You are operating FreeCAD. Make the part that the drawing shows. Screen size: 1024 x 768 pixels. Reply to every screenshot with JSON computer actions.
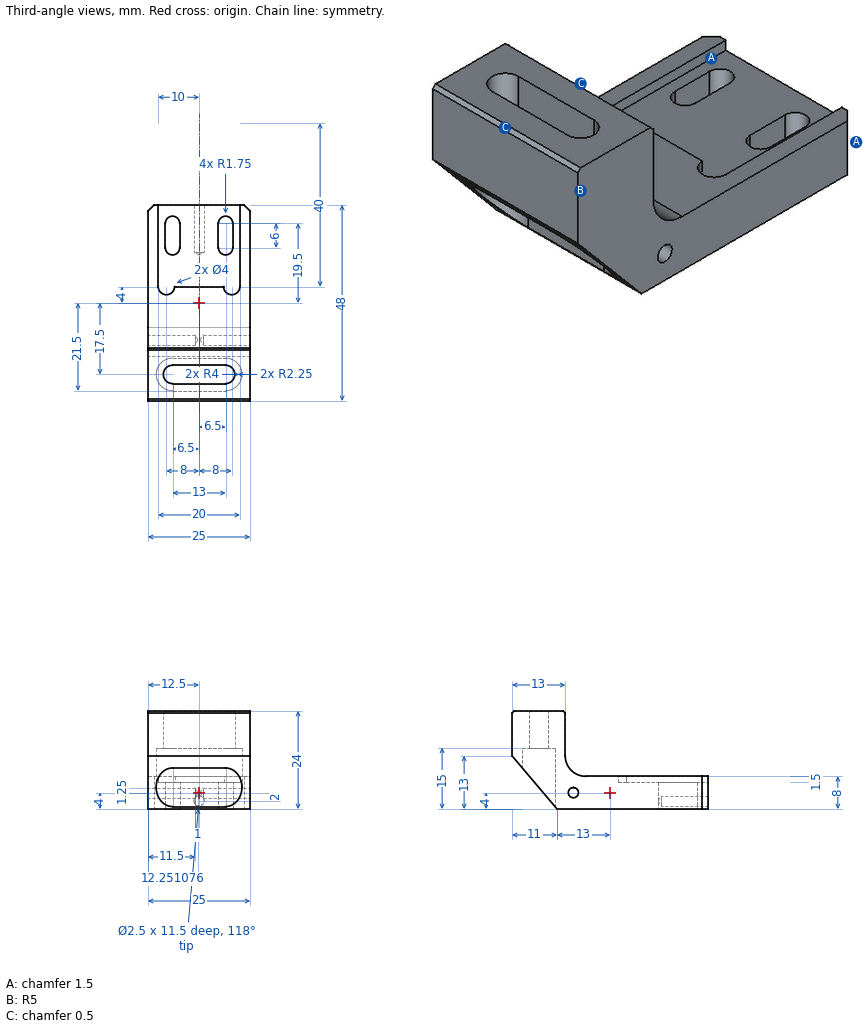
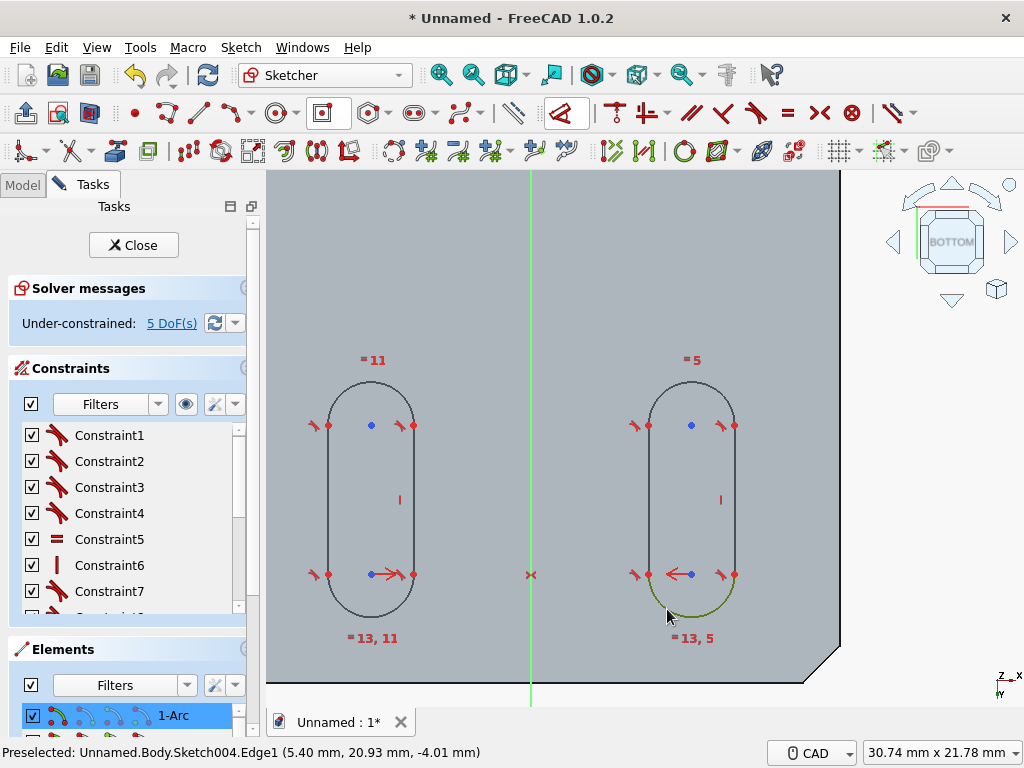
{"action": "left_click", "coordinate": [584, 114]}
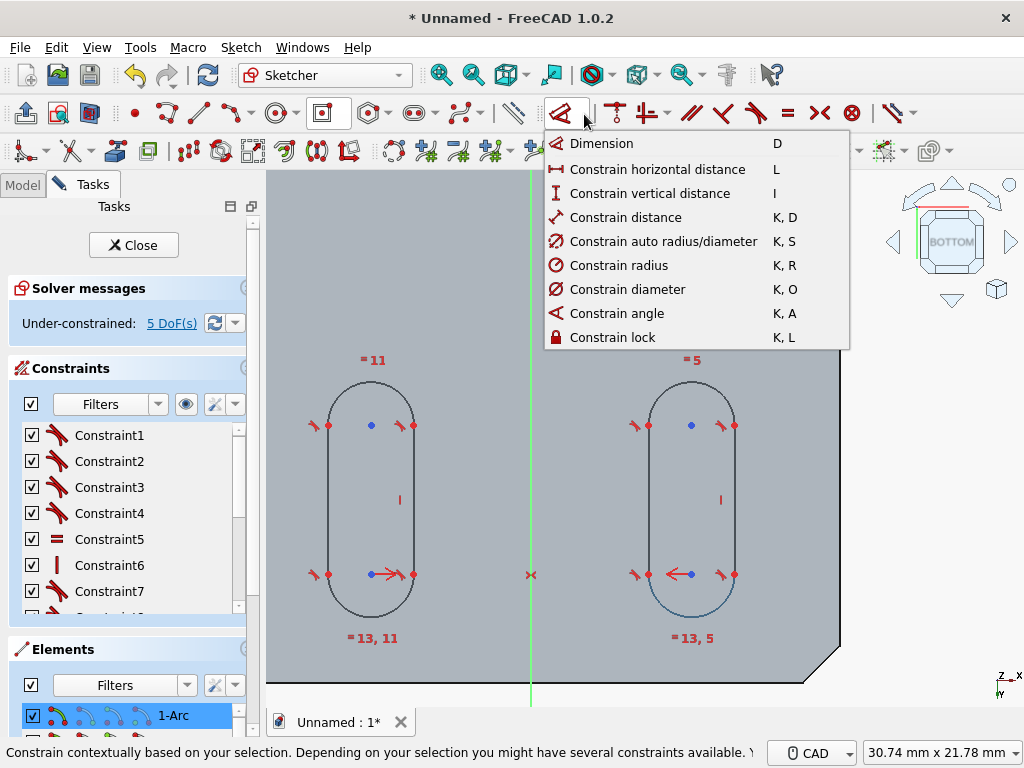
{"action": "left_click", "coordinate": [697, 265]}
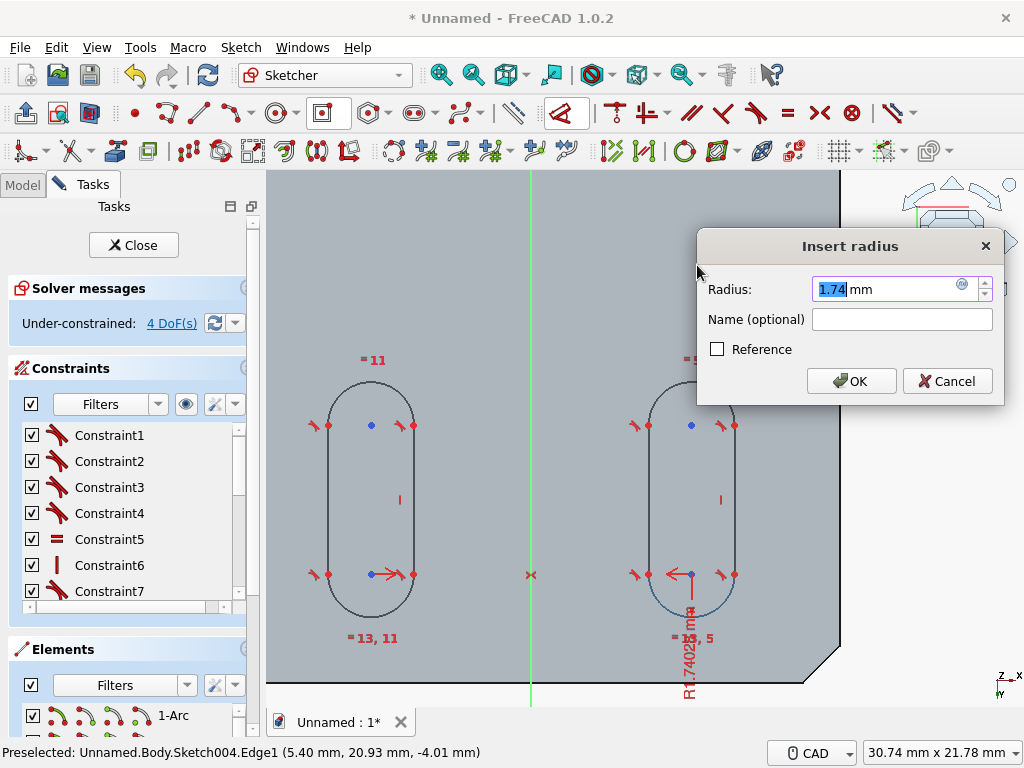
{"action": "type", "text": "1.75"}
{"action": "key", "text": "Return"}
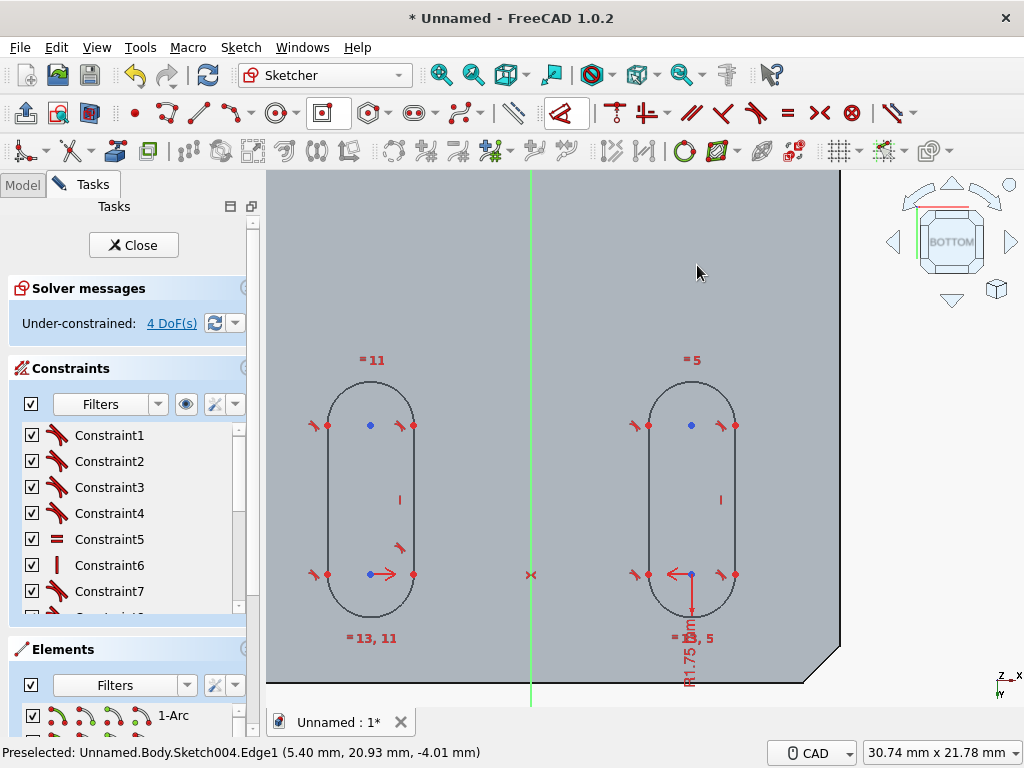
{"action": "left_click", "coordinate": [649, 530]}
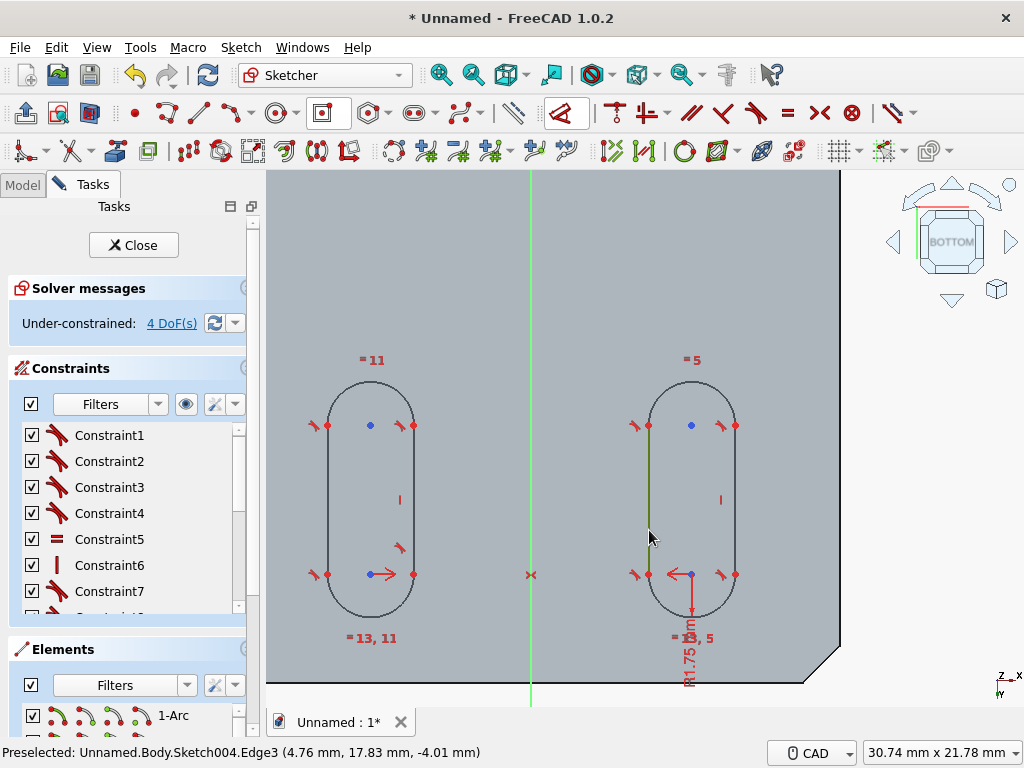
{"action": "left_click", "coordinate": [584, 114]}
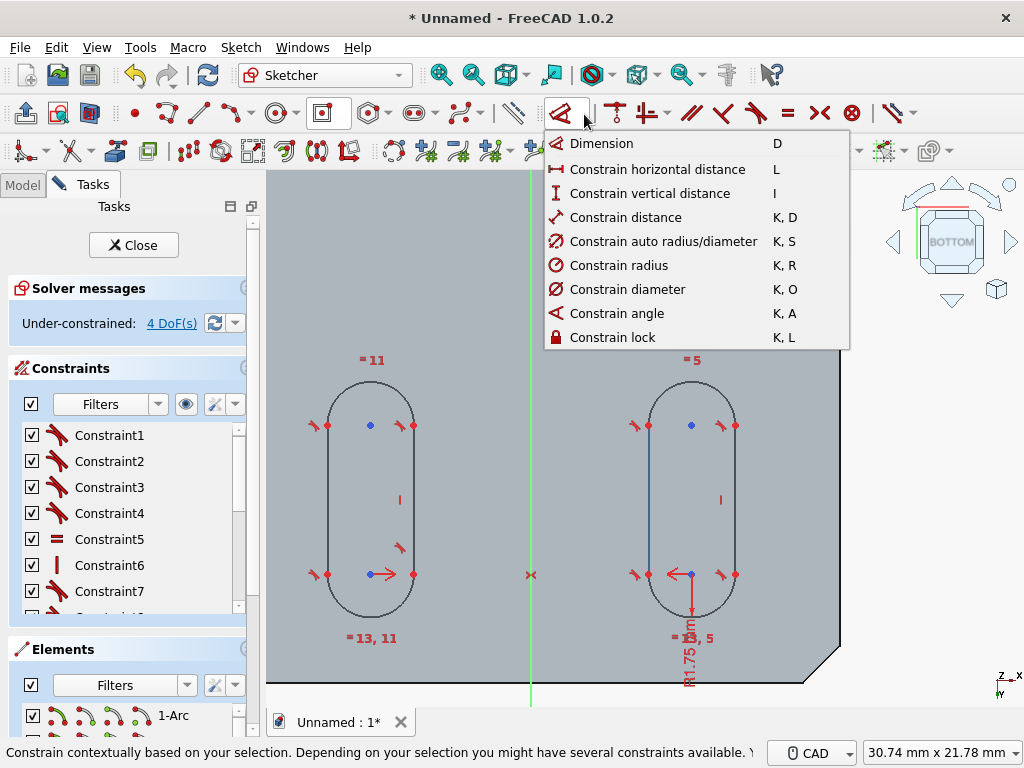
{"action": "left_click", "coordinate": [697, 193]}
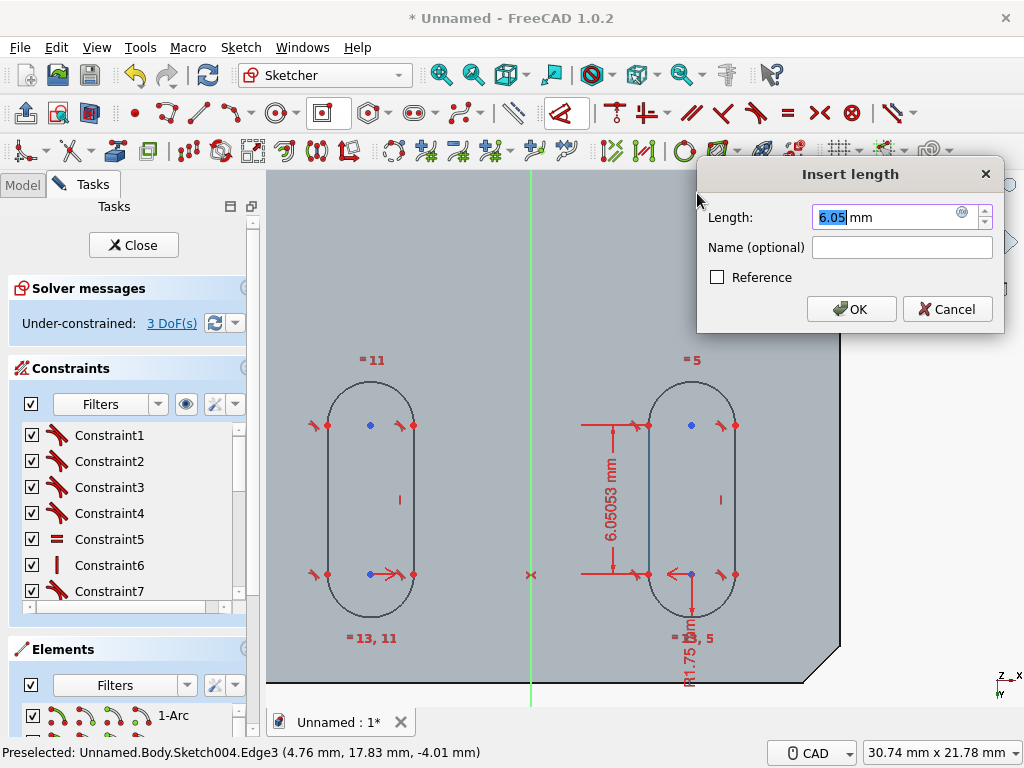
{"action": "type", "text": "6"}
{"action": "key", "text": "Return"}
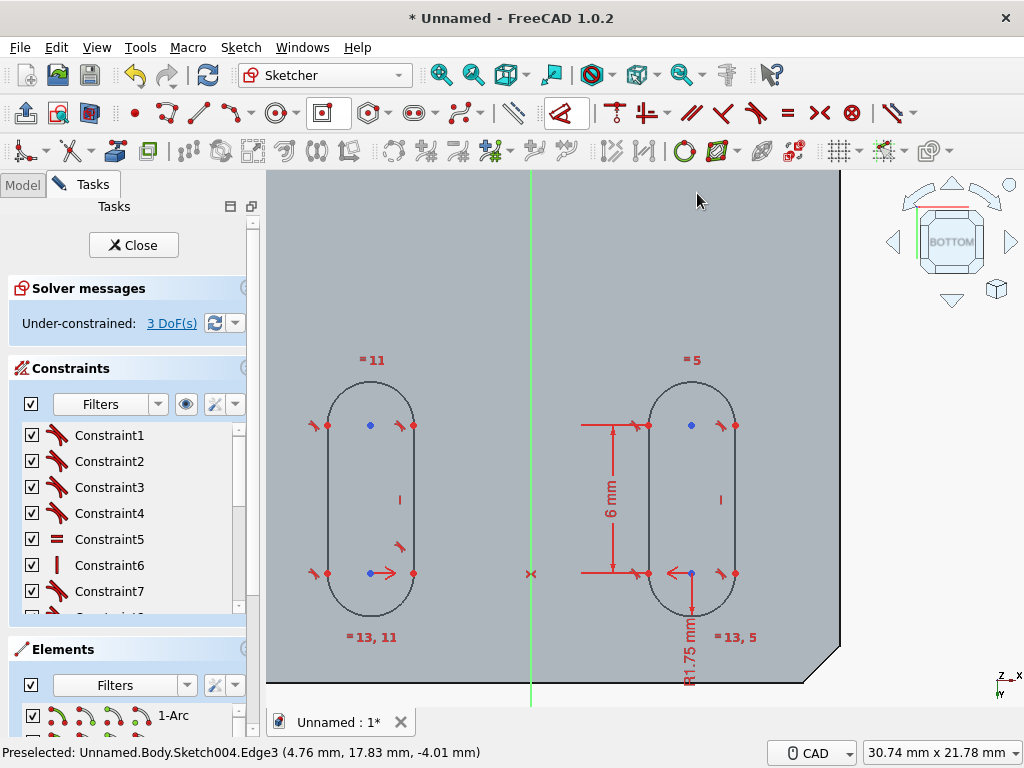
{"action": "left_click", "coordinate": [328, 529]}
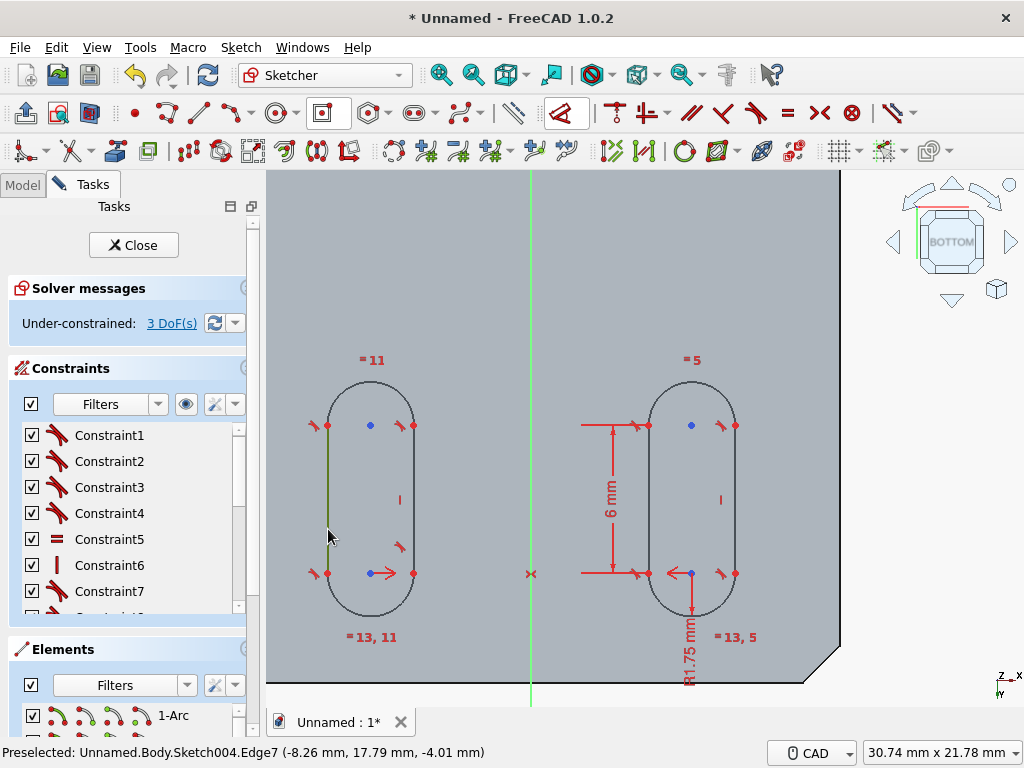
{"action": "key", "text": "i"}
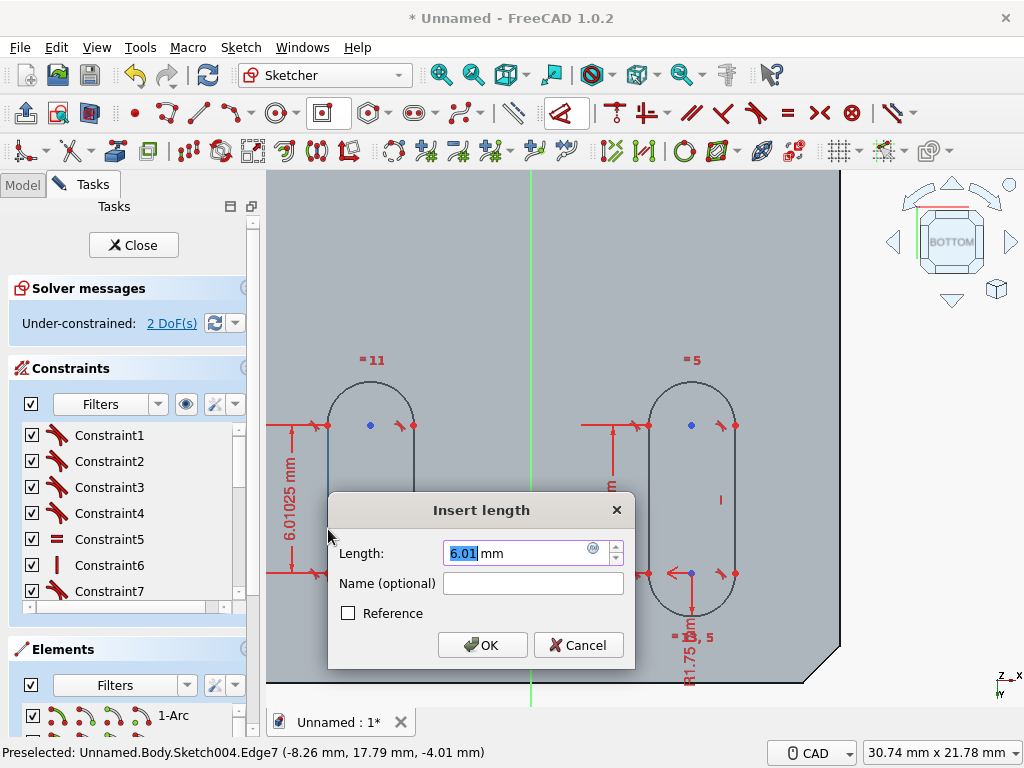
{"action": "type", "text": "6"}
{"action": "key", "text": "Return"}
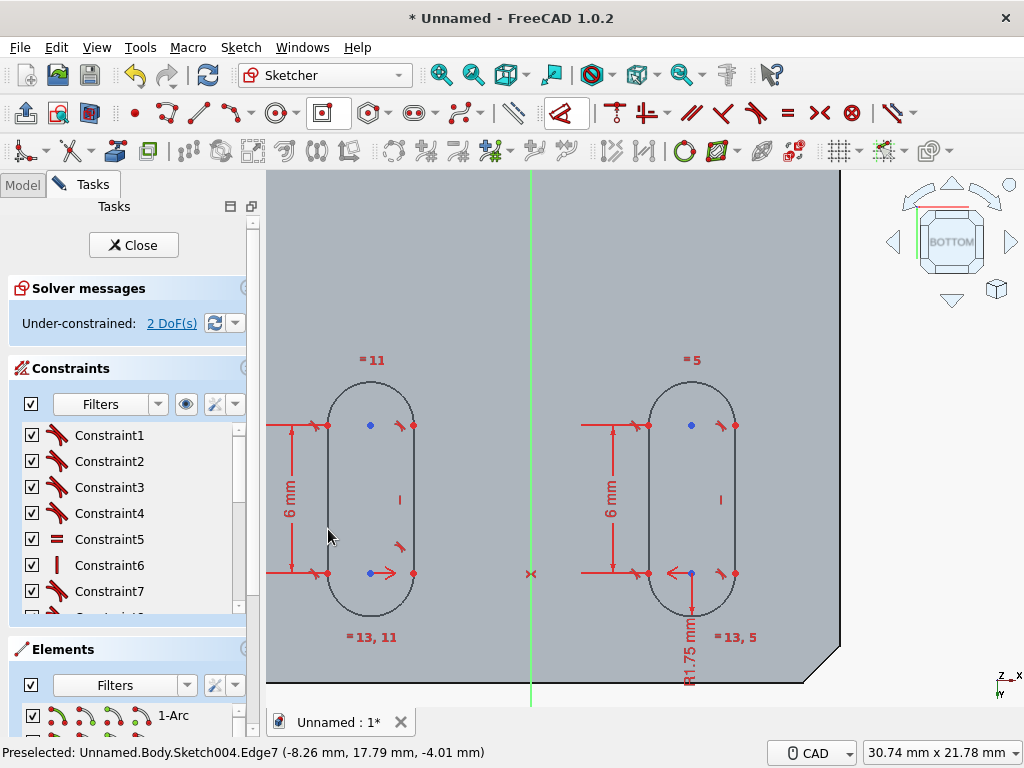
{"action": "left_click", "coordinate": [692, 573]}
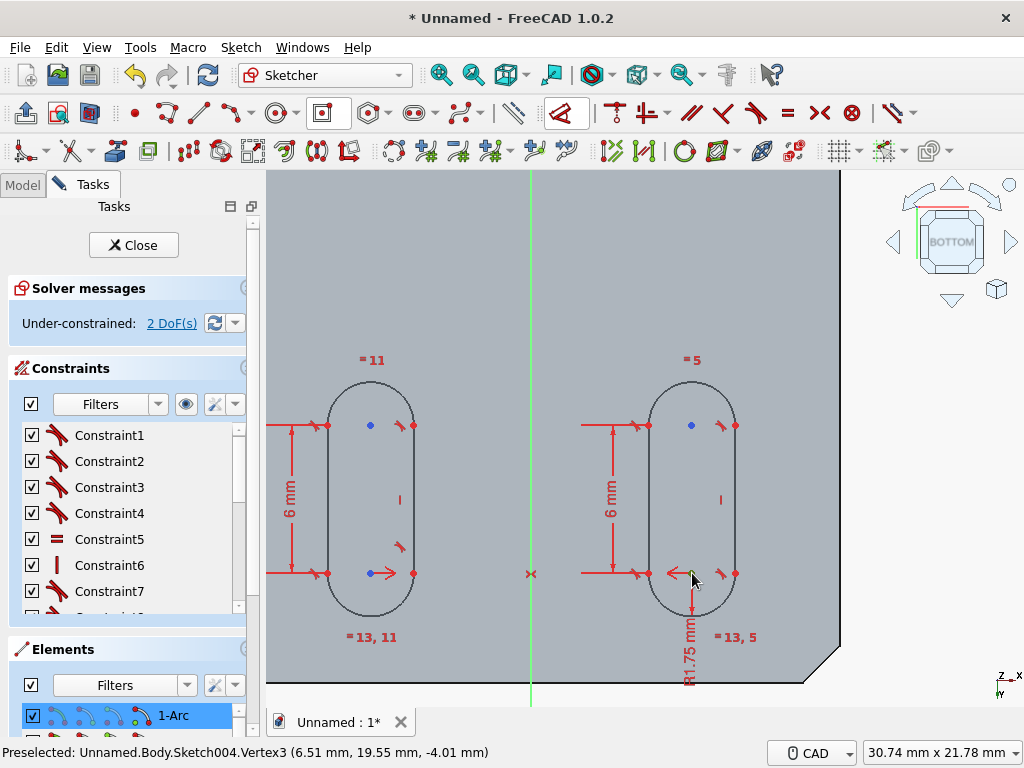
{"action": "left_click", "coordinate": [584, 114]}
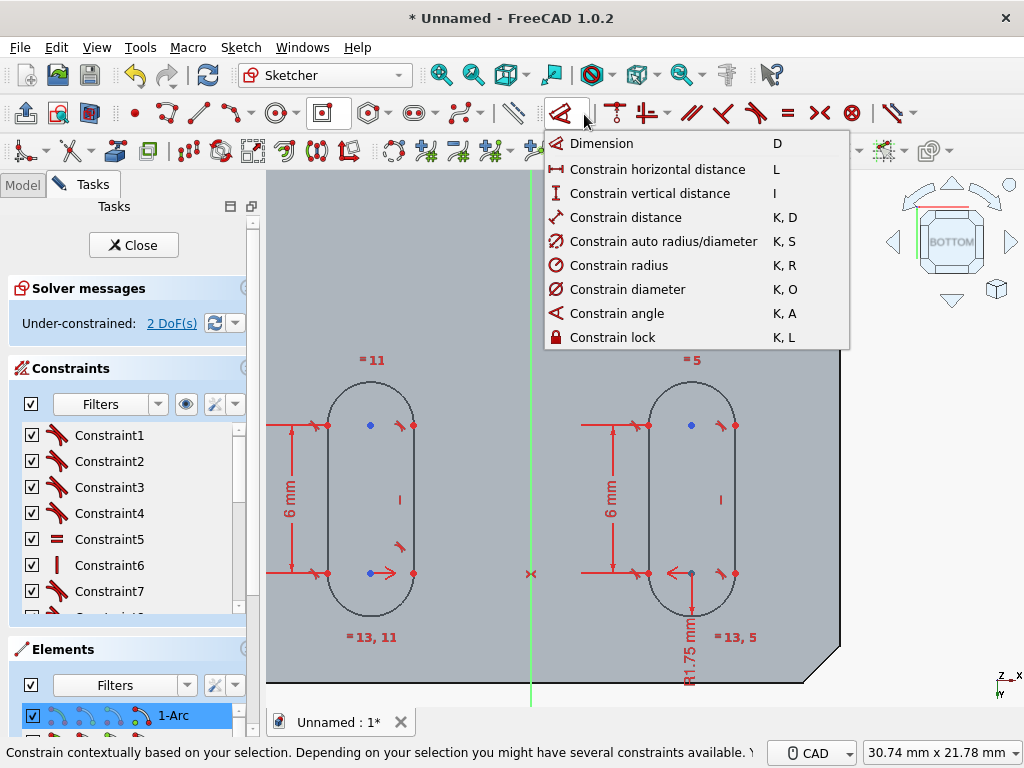
{"action": "left_click", "coordinate": [697, 169]}